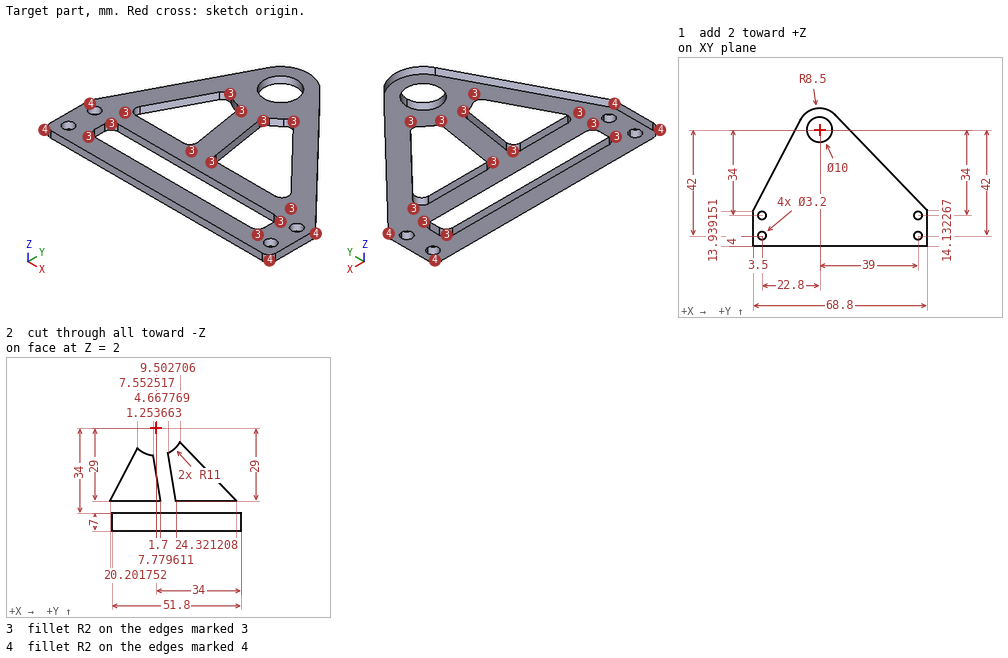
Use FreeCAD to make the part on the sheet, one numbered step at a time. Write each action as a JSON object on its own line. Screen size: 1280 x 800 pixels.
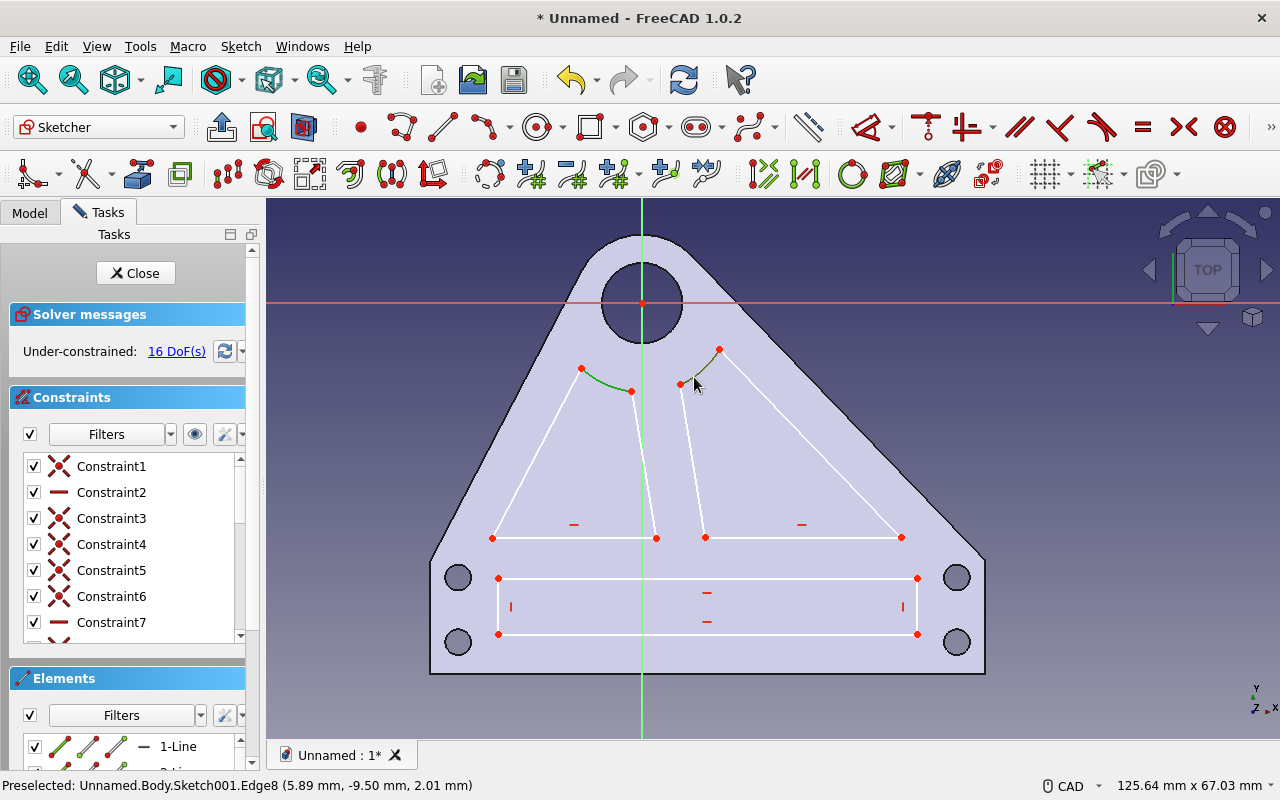
{"action": "left_click", "coordinate": [1143, 128]}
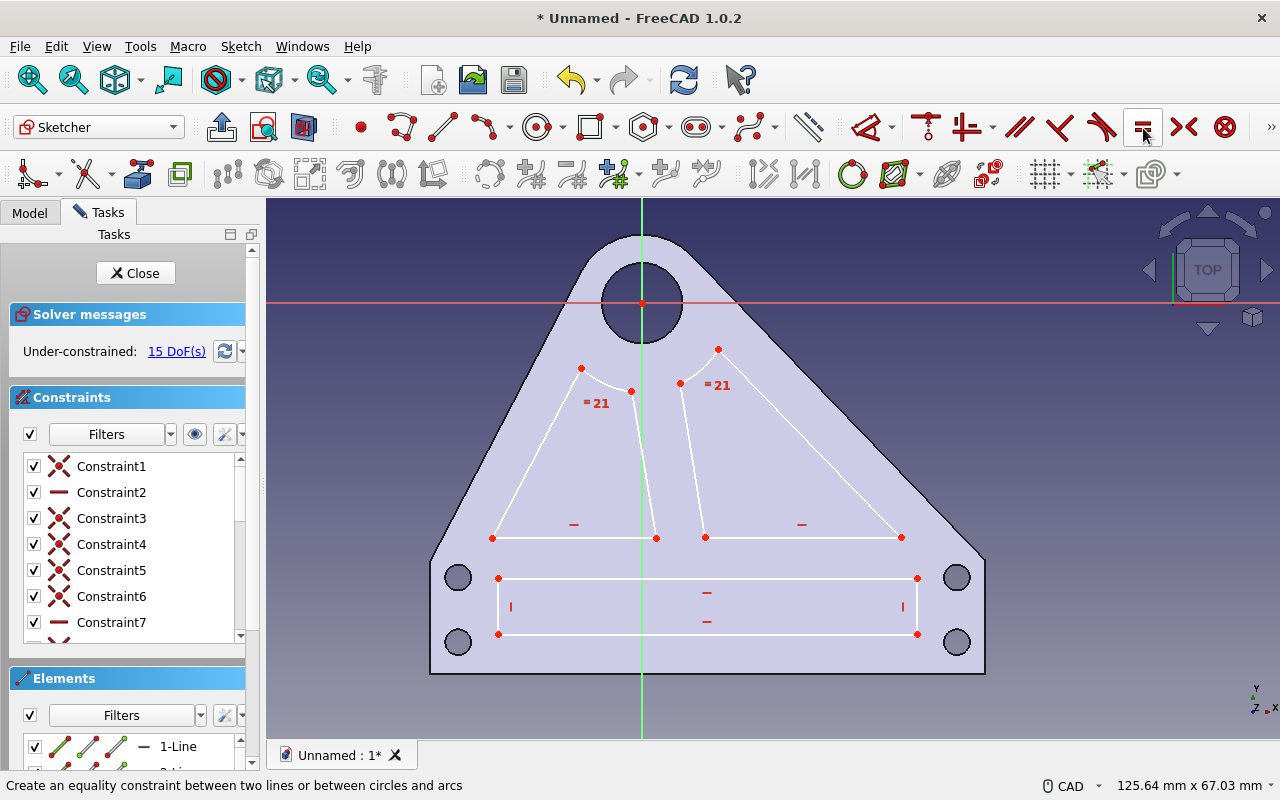
{"action": "left_click", "coordinate": [866, 128]}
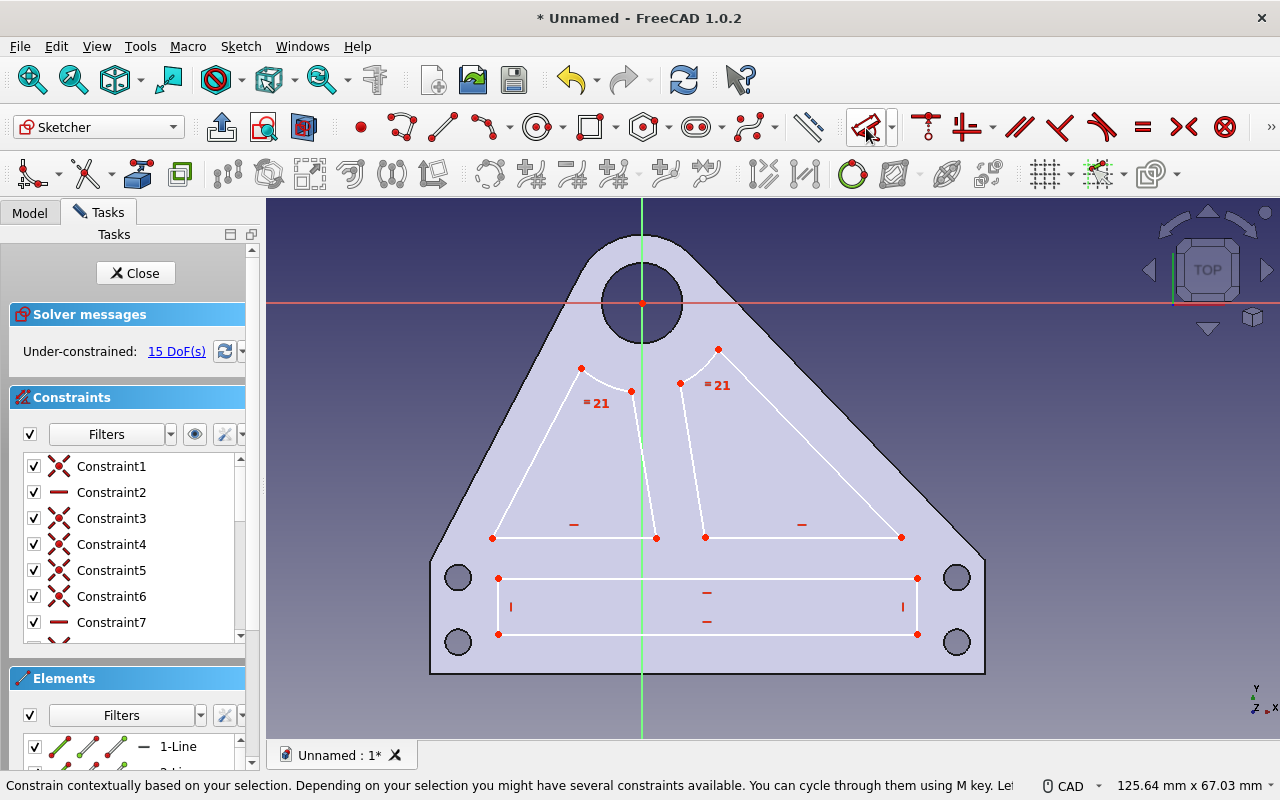
{"action": "left_click", "coordinate": [595, 379]}
{"action": "left_click", "coordinate": [578, 406]}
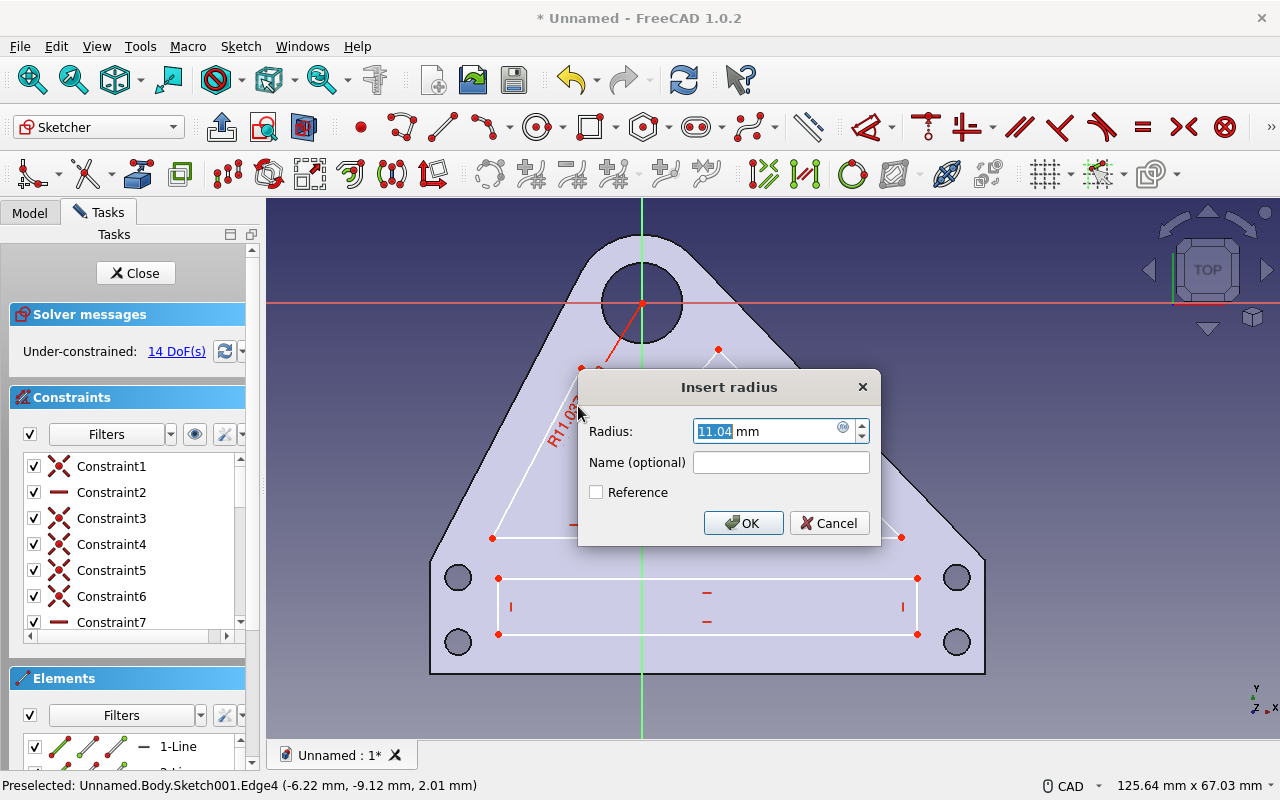
{"action": "type", "text": "11"}
{"action": "key", "text": "Return"}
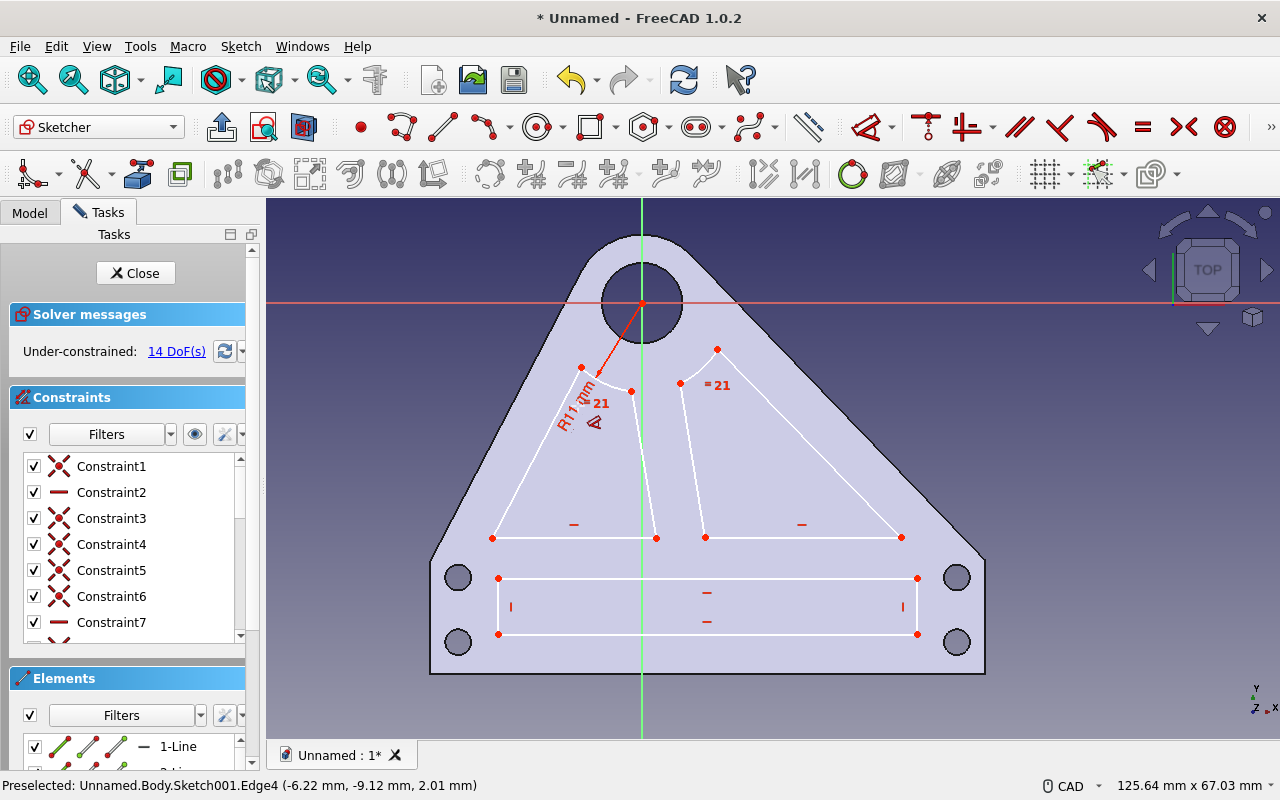
{"action": "left_click", "coordinate": [498, 596]}
{"action": "left_click", "coordinate": [464, 607]}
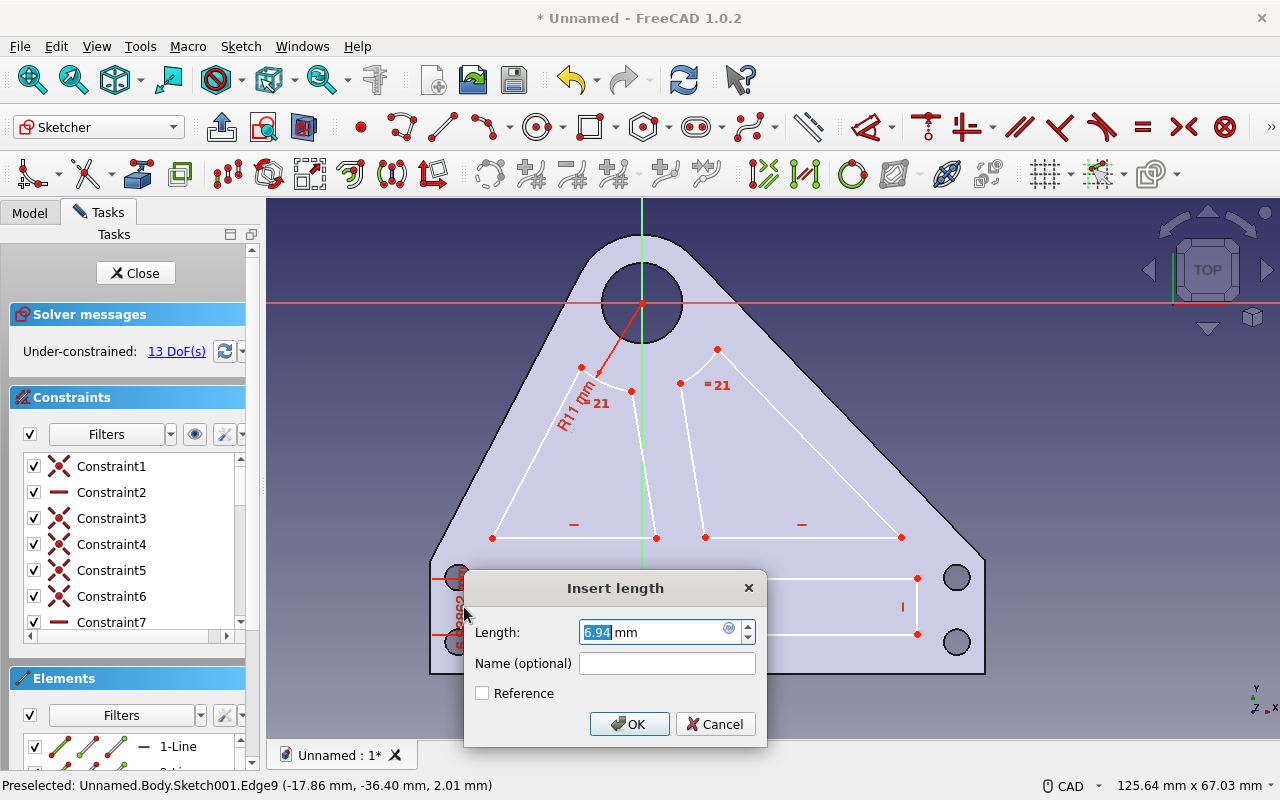
{"action": "type", "text": "7"}
{"action": "key", "text": "Return"}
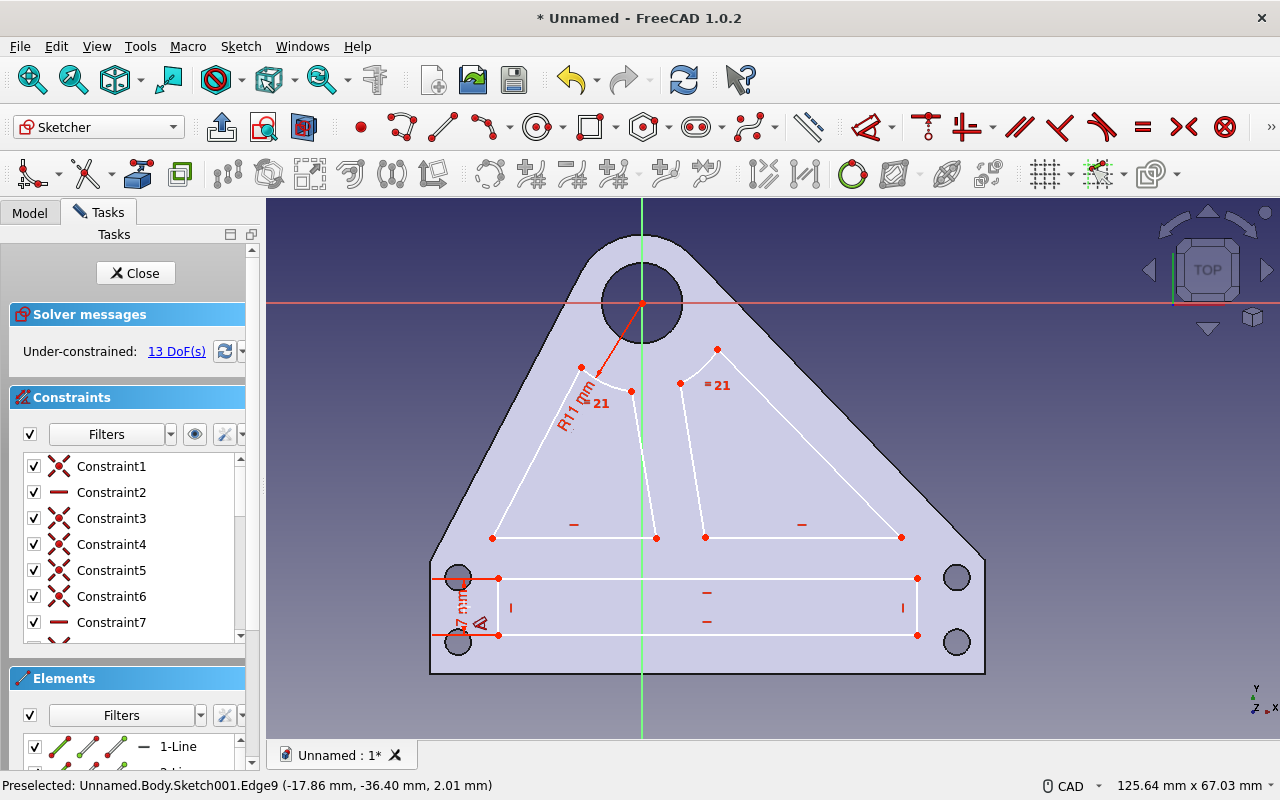
{"action": "left_click", "coordinate": [492, 538]}
{"action": "left_click", "coordinate": [458, 421]}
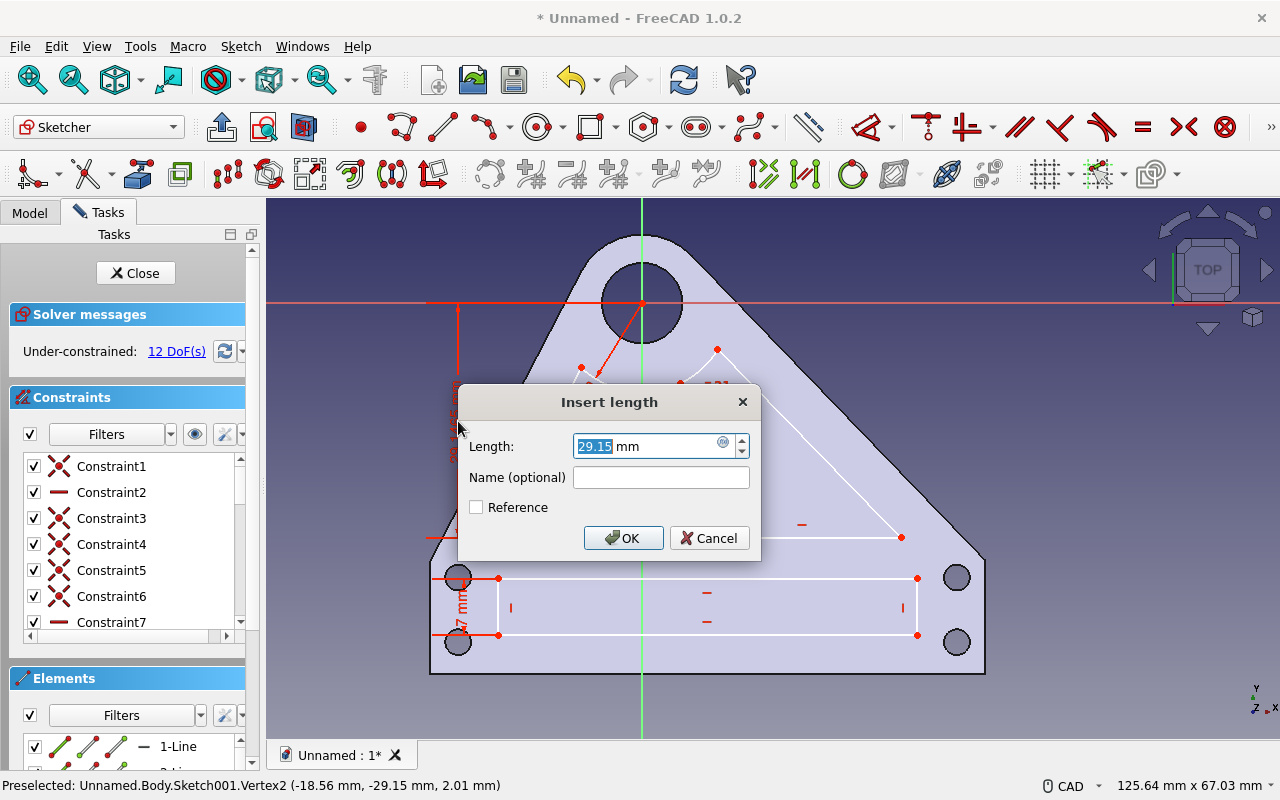
{"action": "type", "text": "29"}
{"action": "key", "text": "Return"}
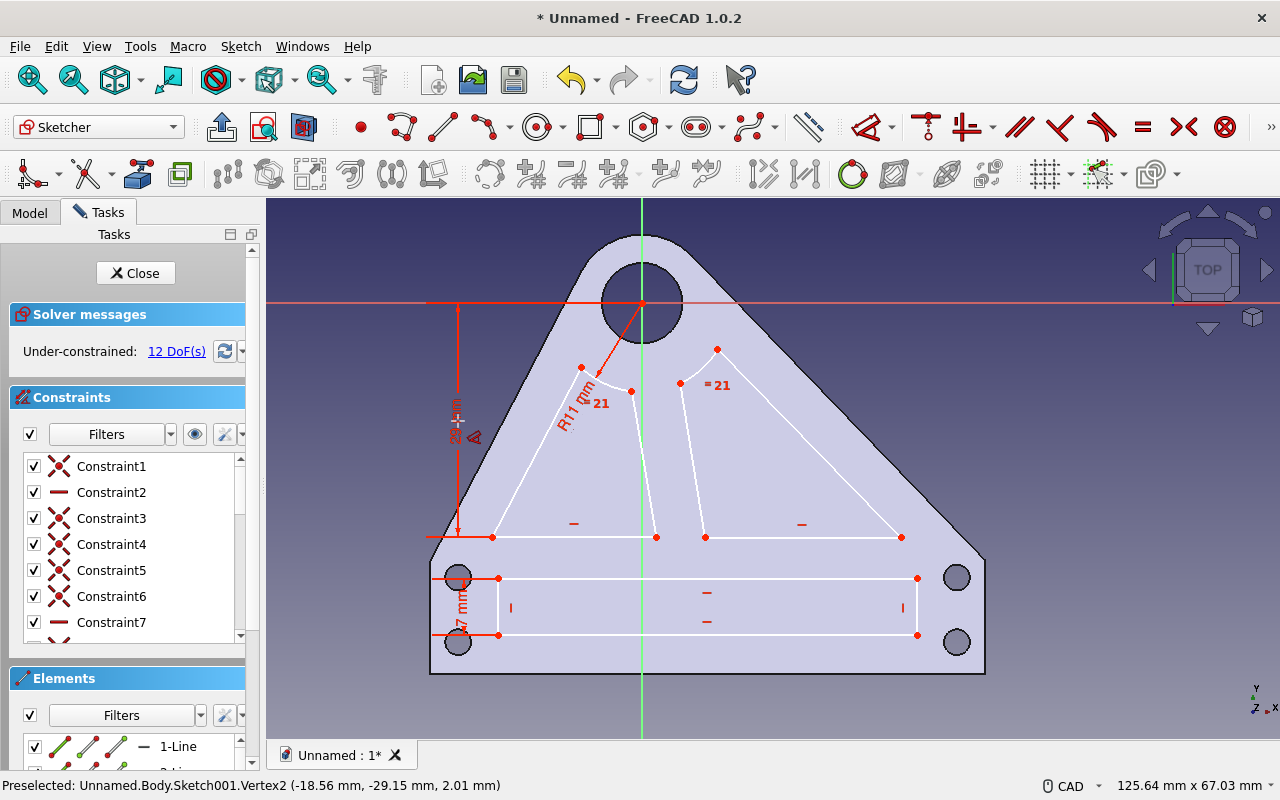
{"action": "left_click", "coordinate": [705, 538]}
{"action": "left_click", "coordinate": [608, 367]}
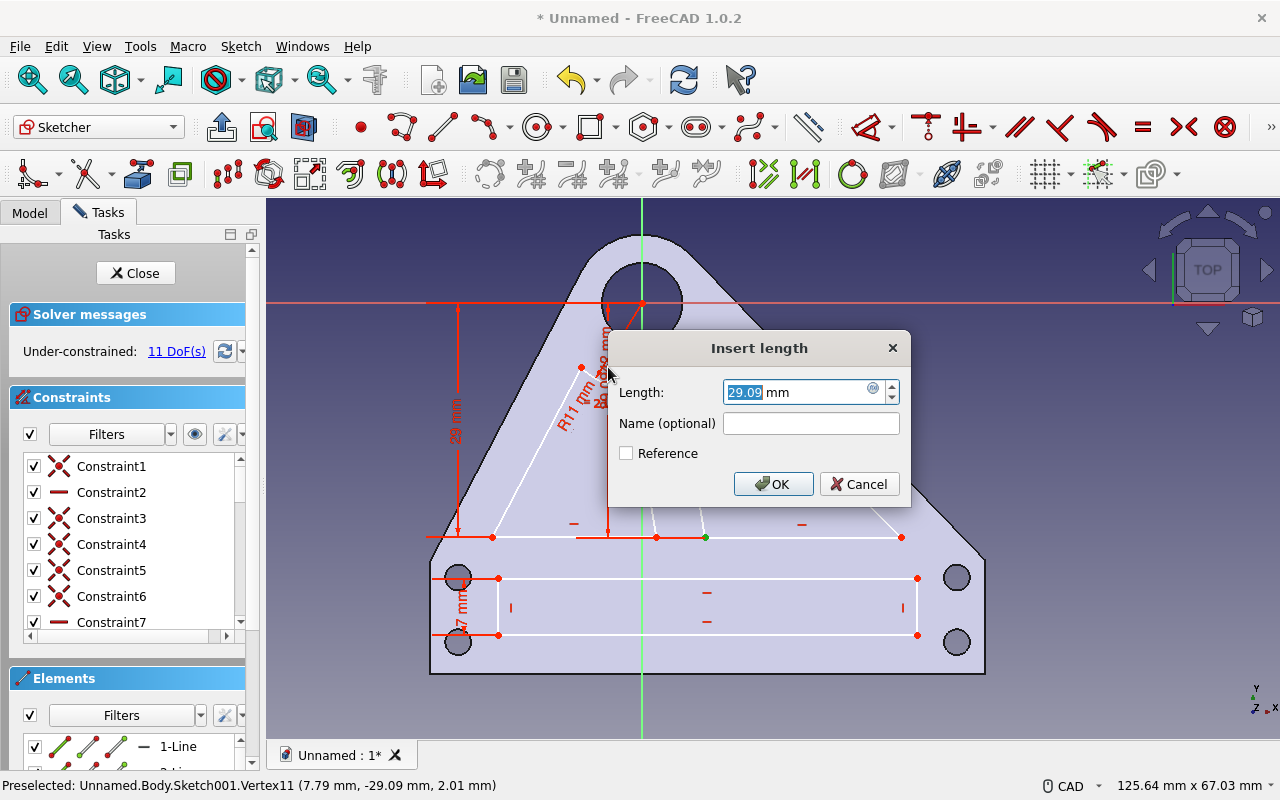
{"action": "type", "text": "29"}
{"action": "key", "text": "Return"}